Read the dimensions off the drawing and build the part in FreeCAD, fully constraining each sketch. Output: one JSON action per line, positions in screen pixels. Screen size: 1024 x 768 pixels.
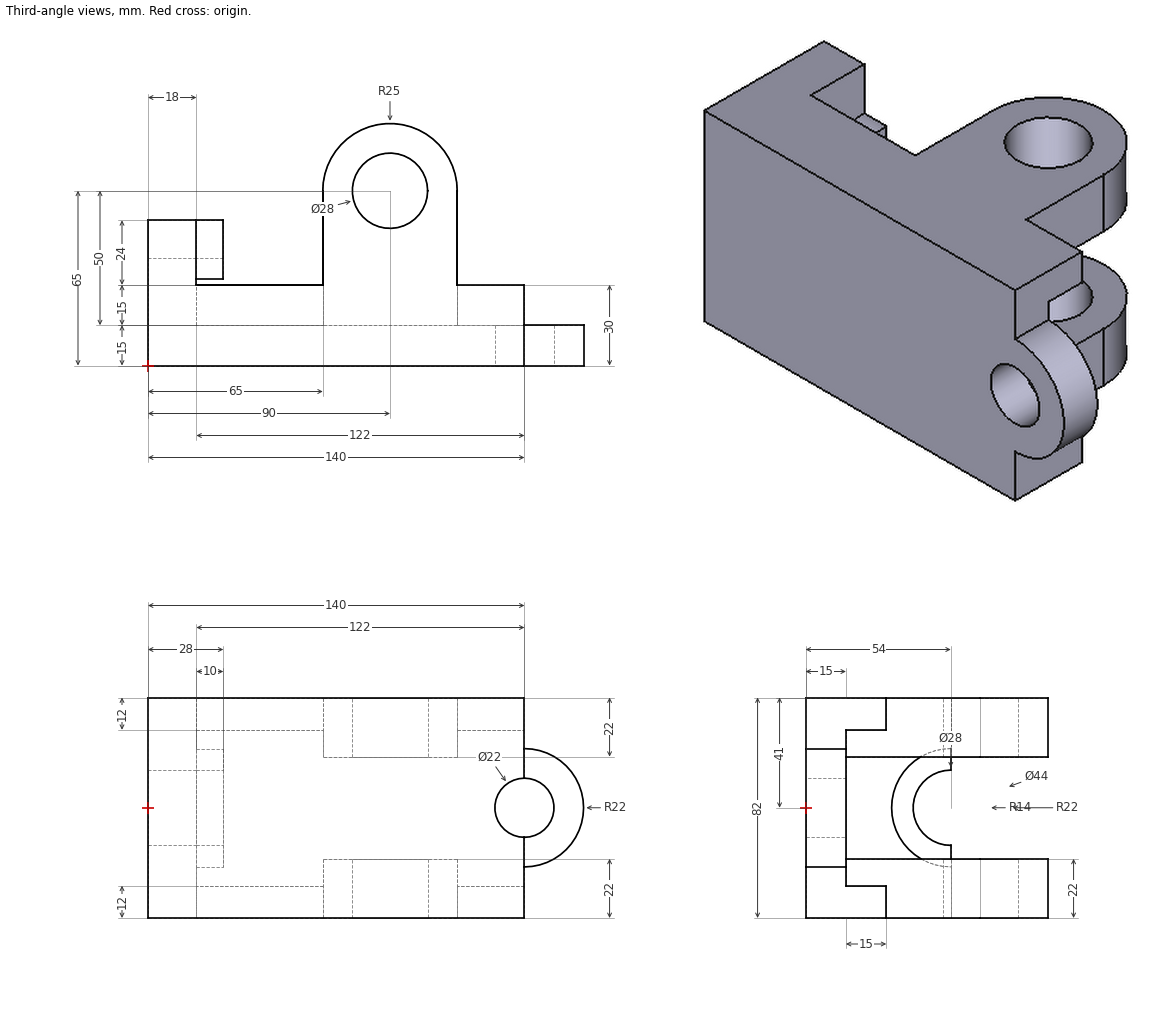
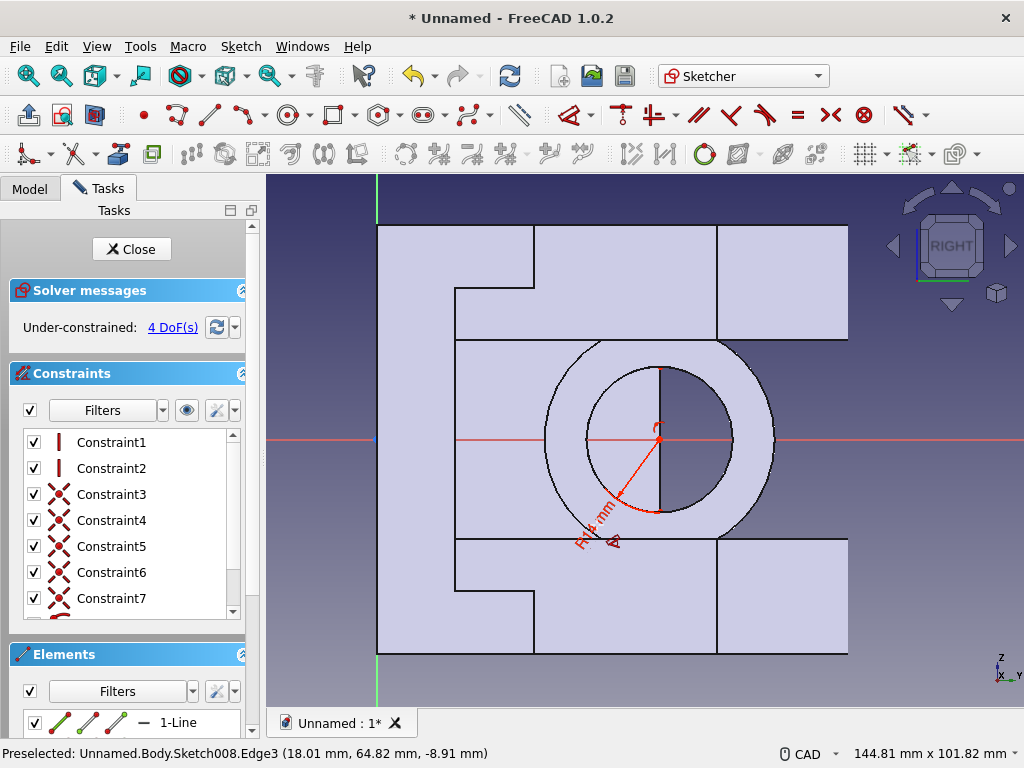
{"action": "left_click", "coordinate": [753, 507]}
{"action": "left_click", "coordinate": [779, 526]}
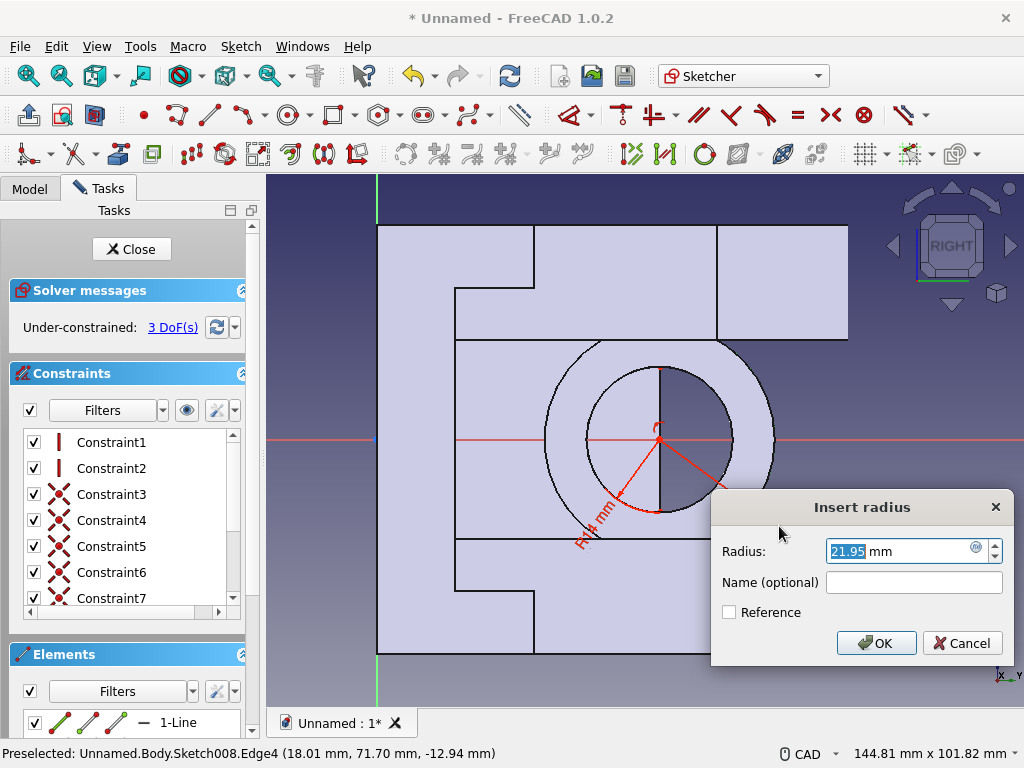
{"action": "type", "text": "22"}
{"action": "key", "text": "Return"}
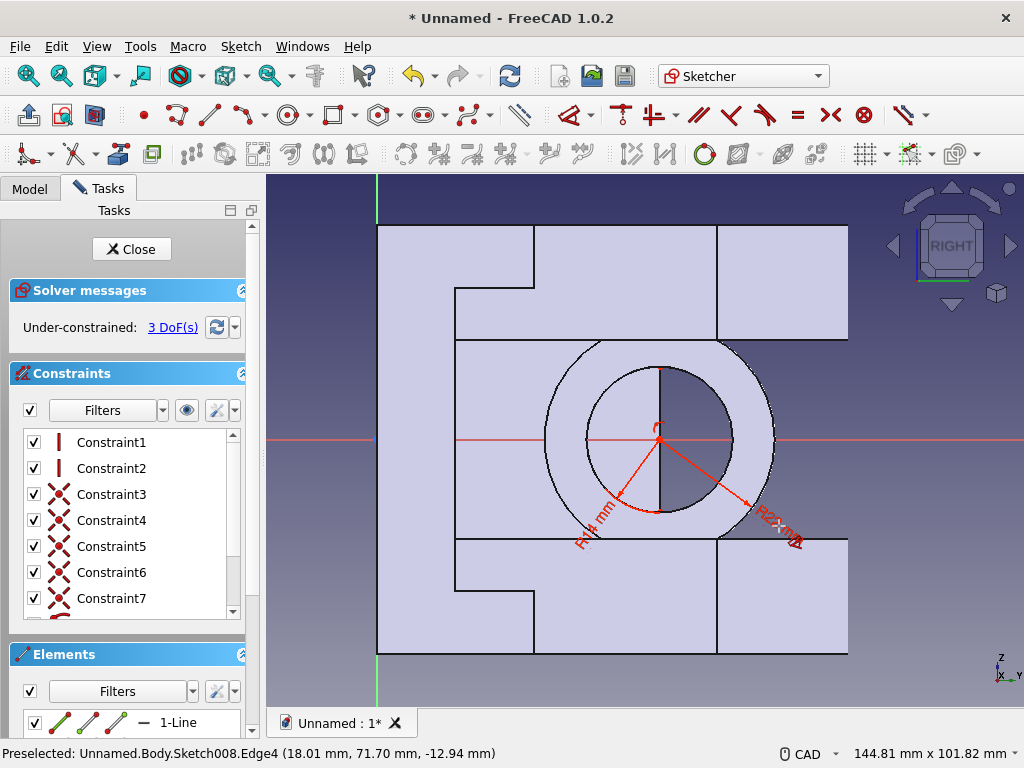
{"action": "left_click", "coordinate": [660, 325]}
{"action": "left_click", "coordinate": [518, 291]}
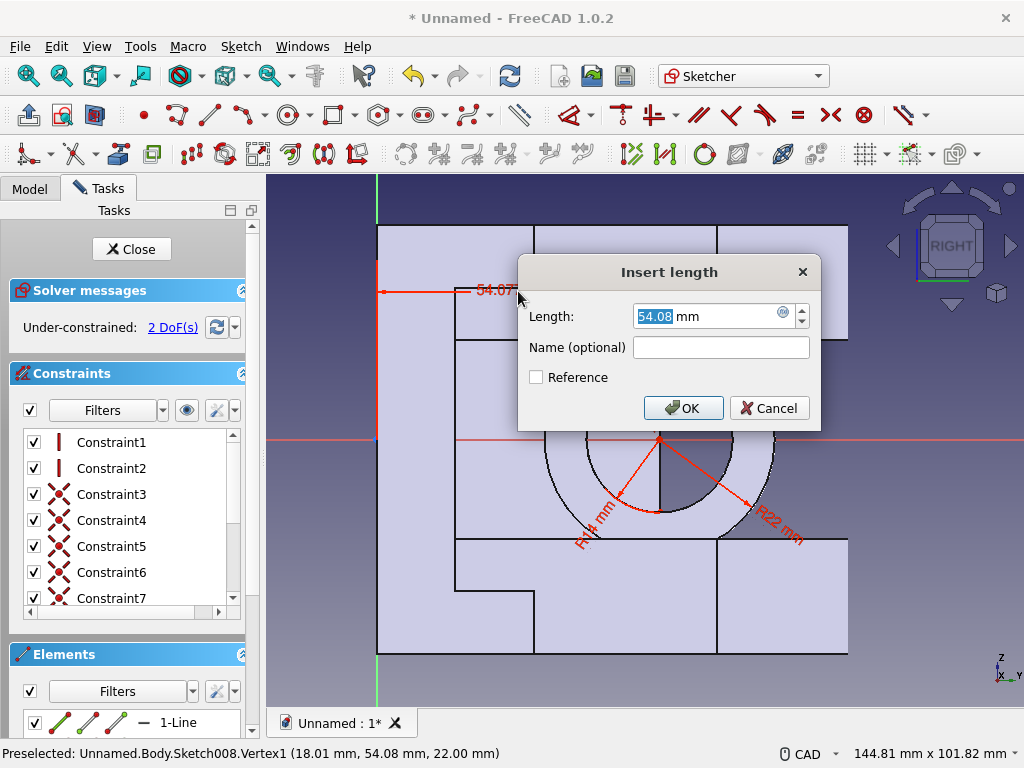
{"action": "type", "text": "54"}
{"action": "key", "text": "Return"}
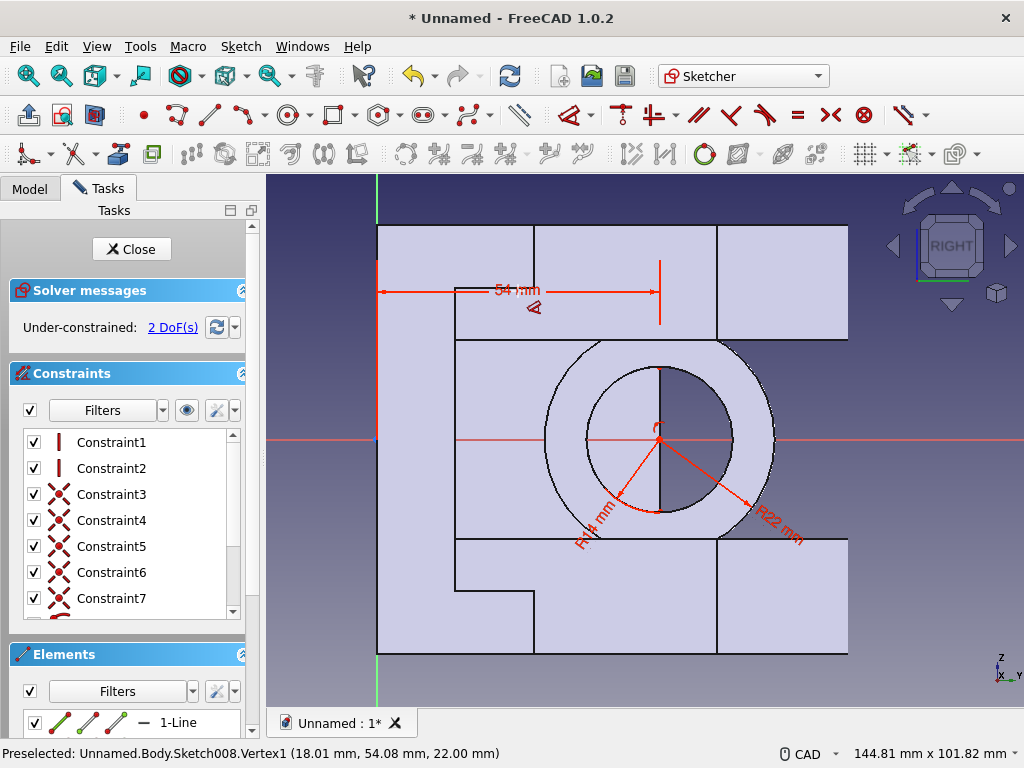
{"action": "left_click", "coordinate": [660, 513]}
{"action": "left_click", "coordinate": [518, 547]}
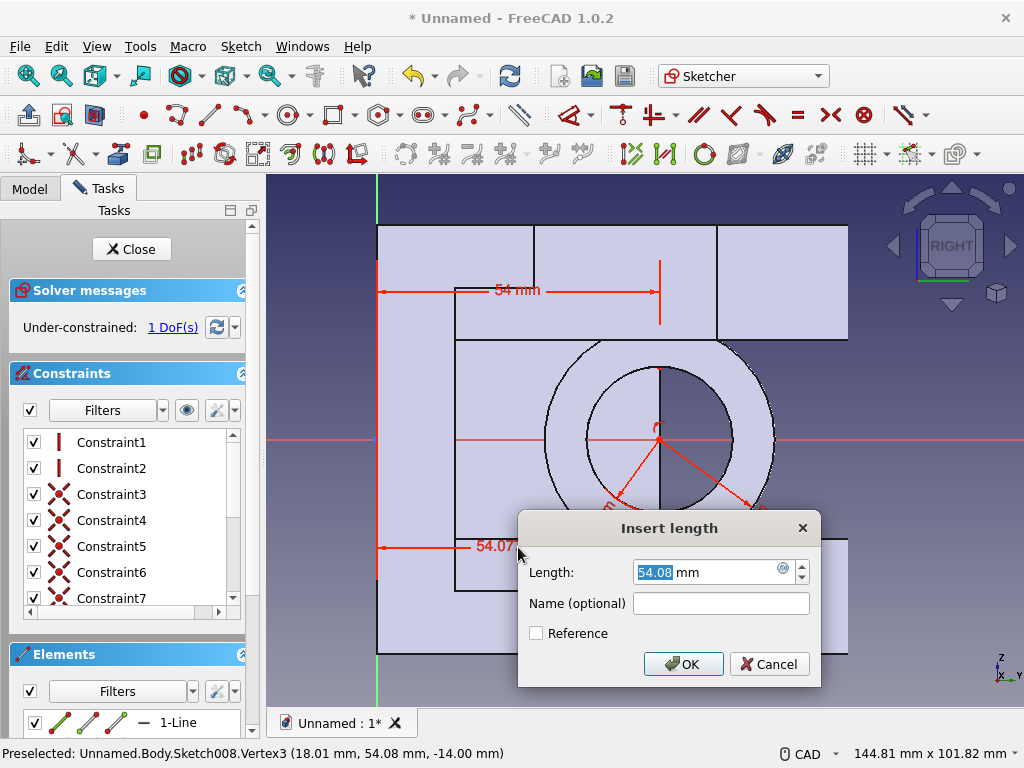
{"action": "type", "text": "54"}
{"action": "key", "text": "Return"}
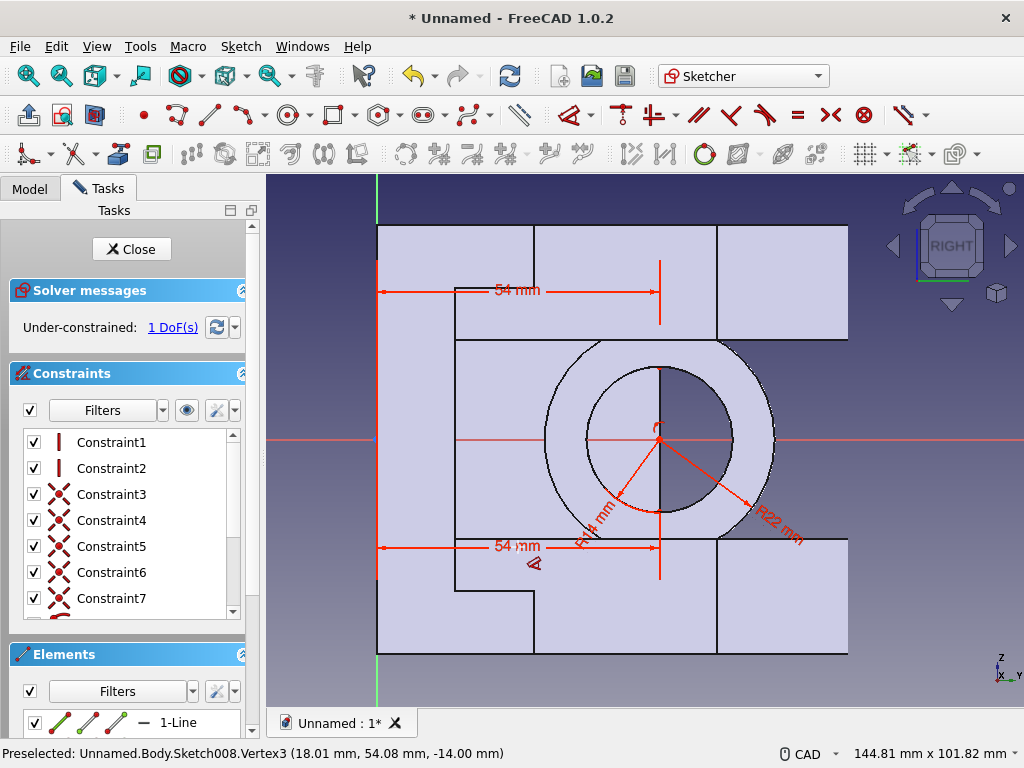
{"action": "left_click", "coordinate": [659, 440]}
{"action": "left_click", "coordinate": [518, 474]}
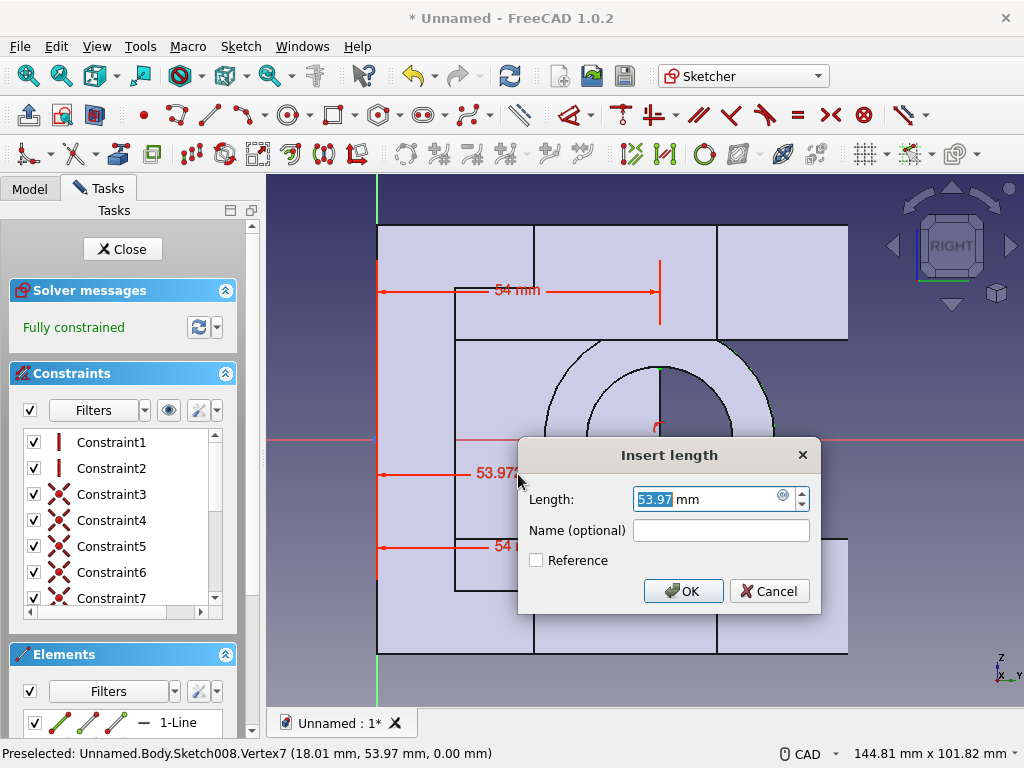
{"action": "type", "text": "54"}
{"action": "key", "text": "Return"}
{"action": "key", "text": "Escape"}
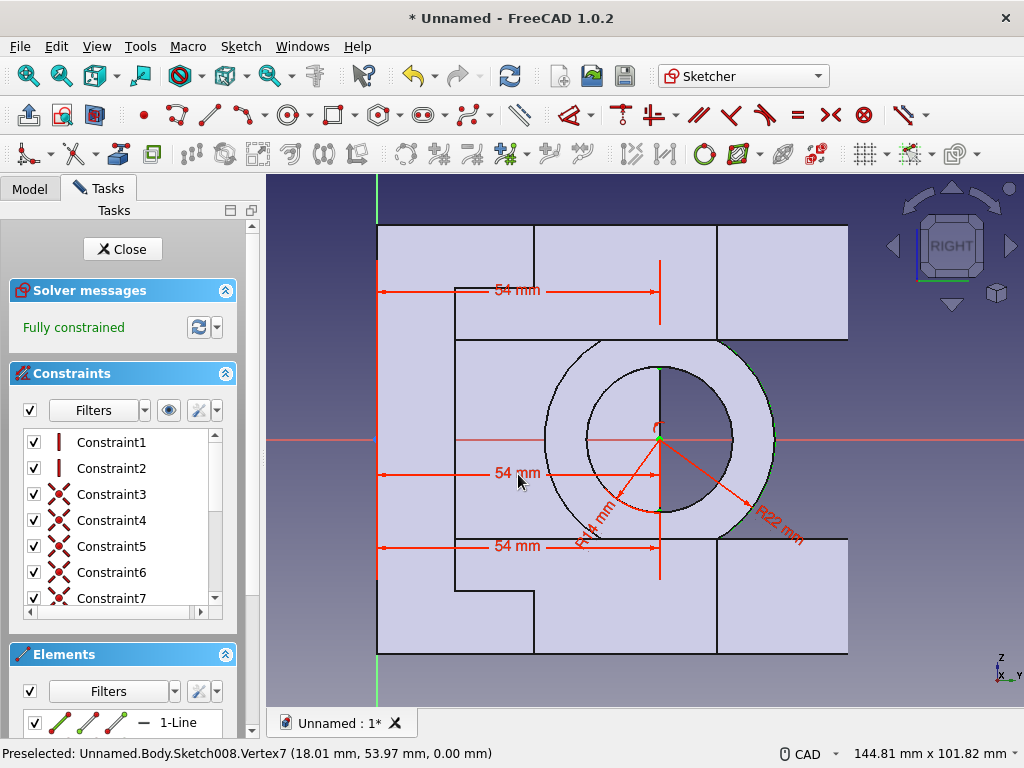
{"action": "left_click", "coordinate": [123, 249]}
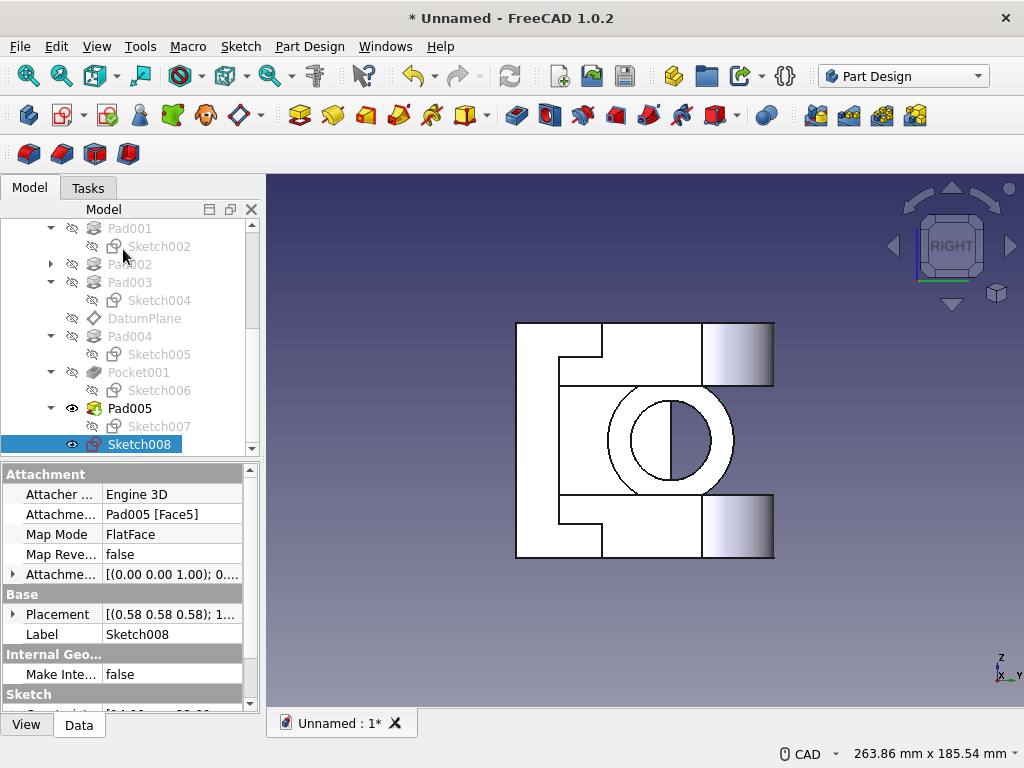
{"action": "left_click", "coordinate": [517, 116]}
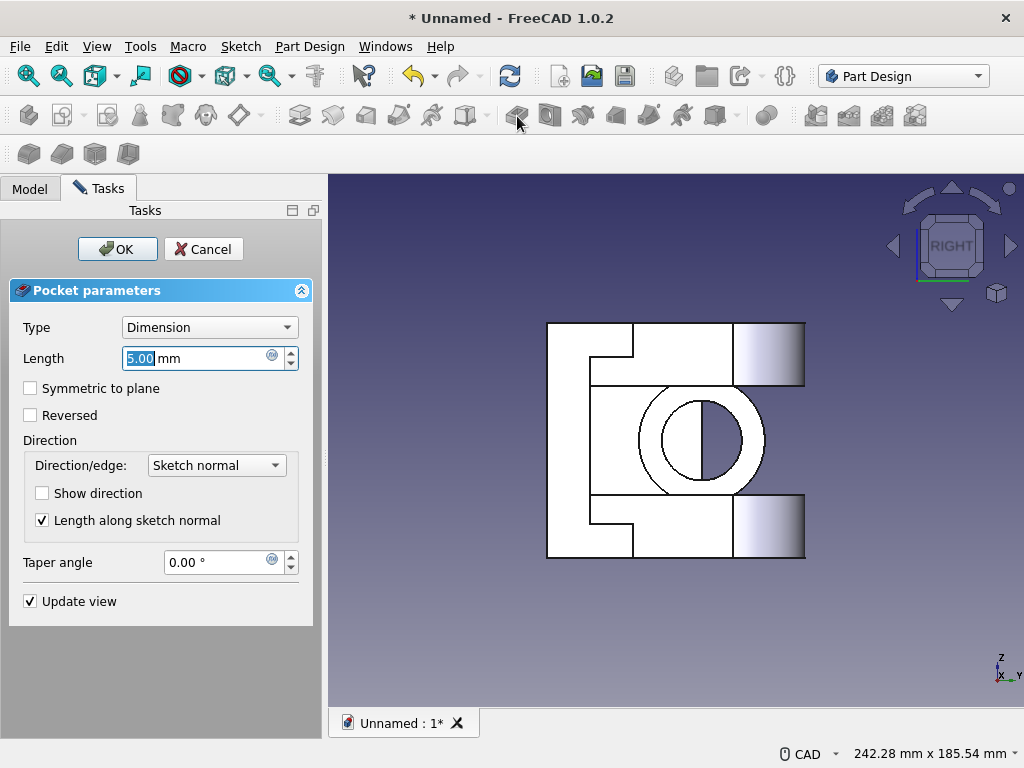
{"action": "type", "text": "10"}
{"action": "key", "text": "Tab"}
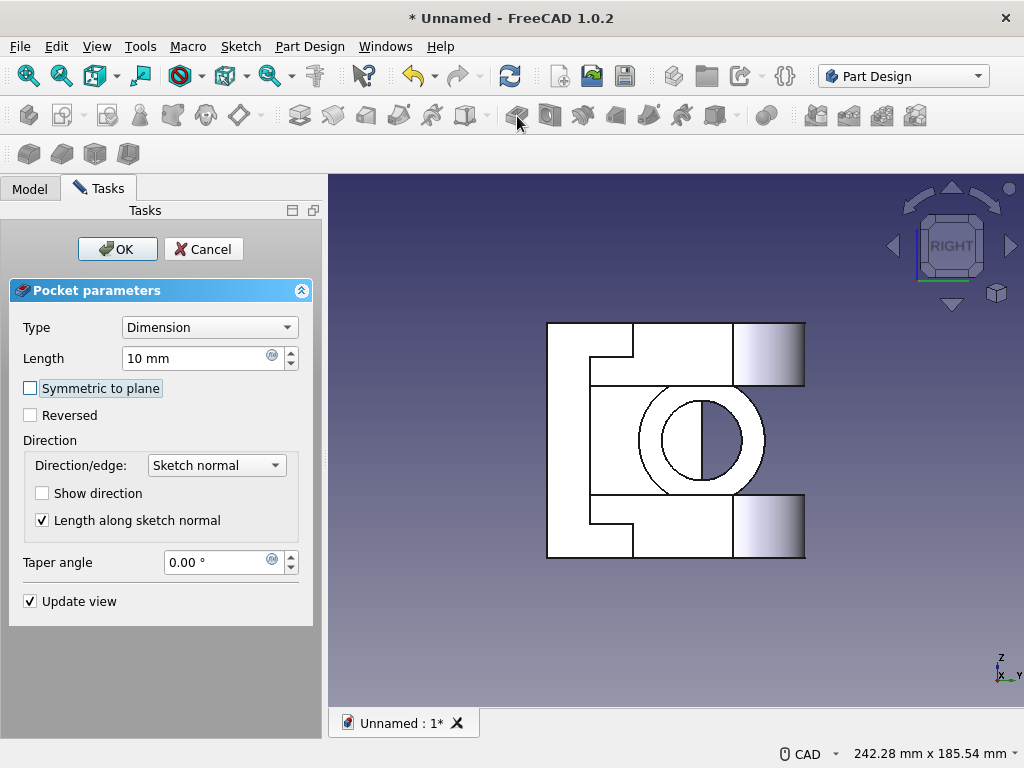
{"action": "left_click", "coordinate": [31, 415]}